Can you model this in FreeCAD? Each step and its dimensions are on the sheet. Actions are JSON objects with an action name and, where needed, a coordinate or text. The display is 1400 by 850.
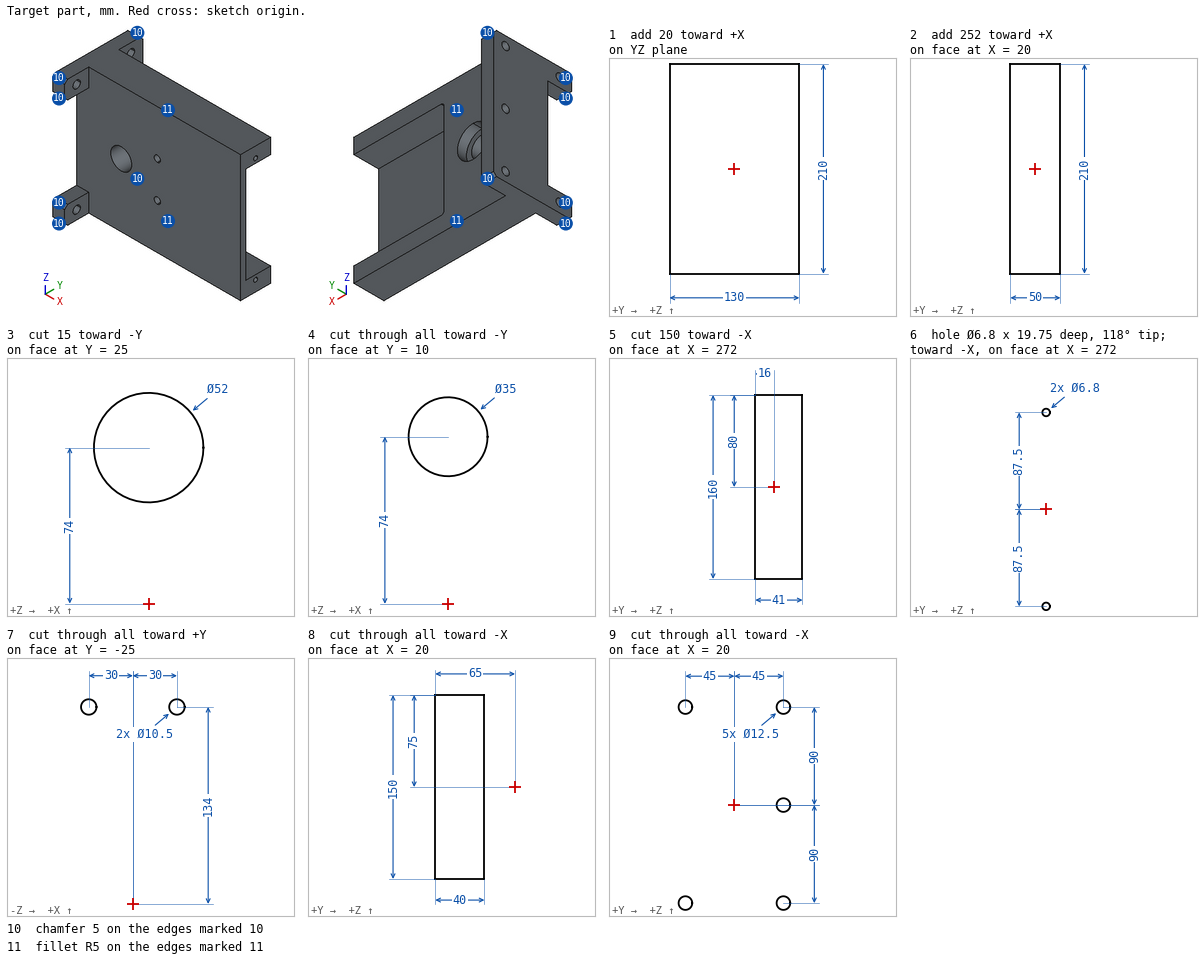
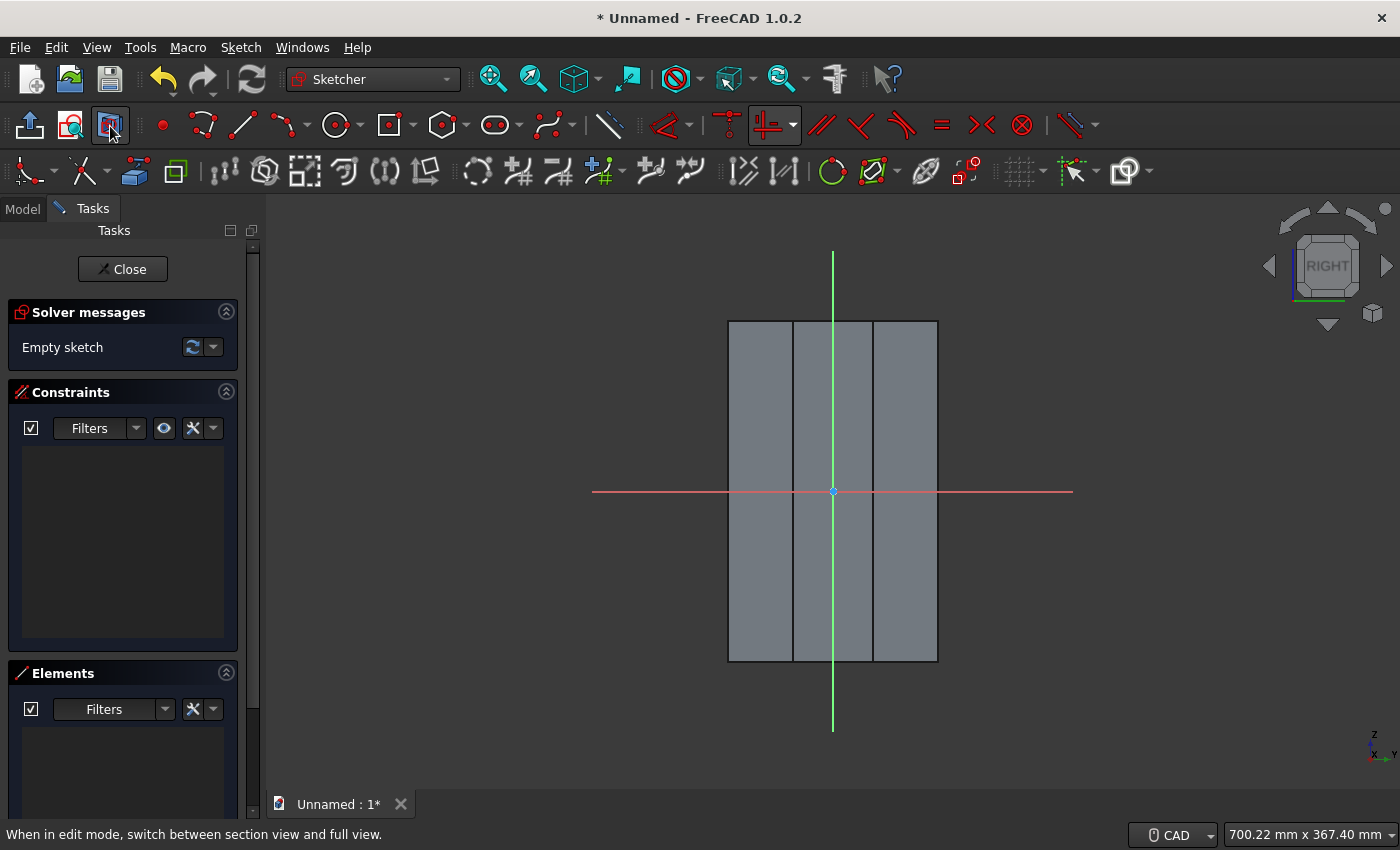
{"action": "scroll", "coordinate": [813, 492], "scroll_direction": "up", "scroll_amount": 2}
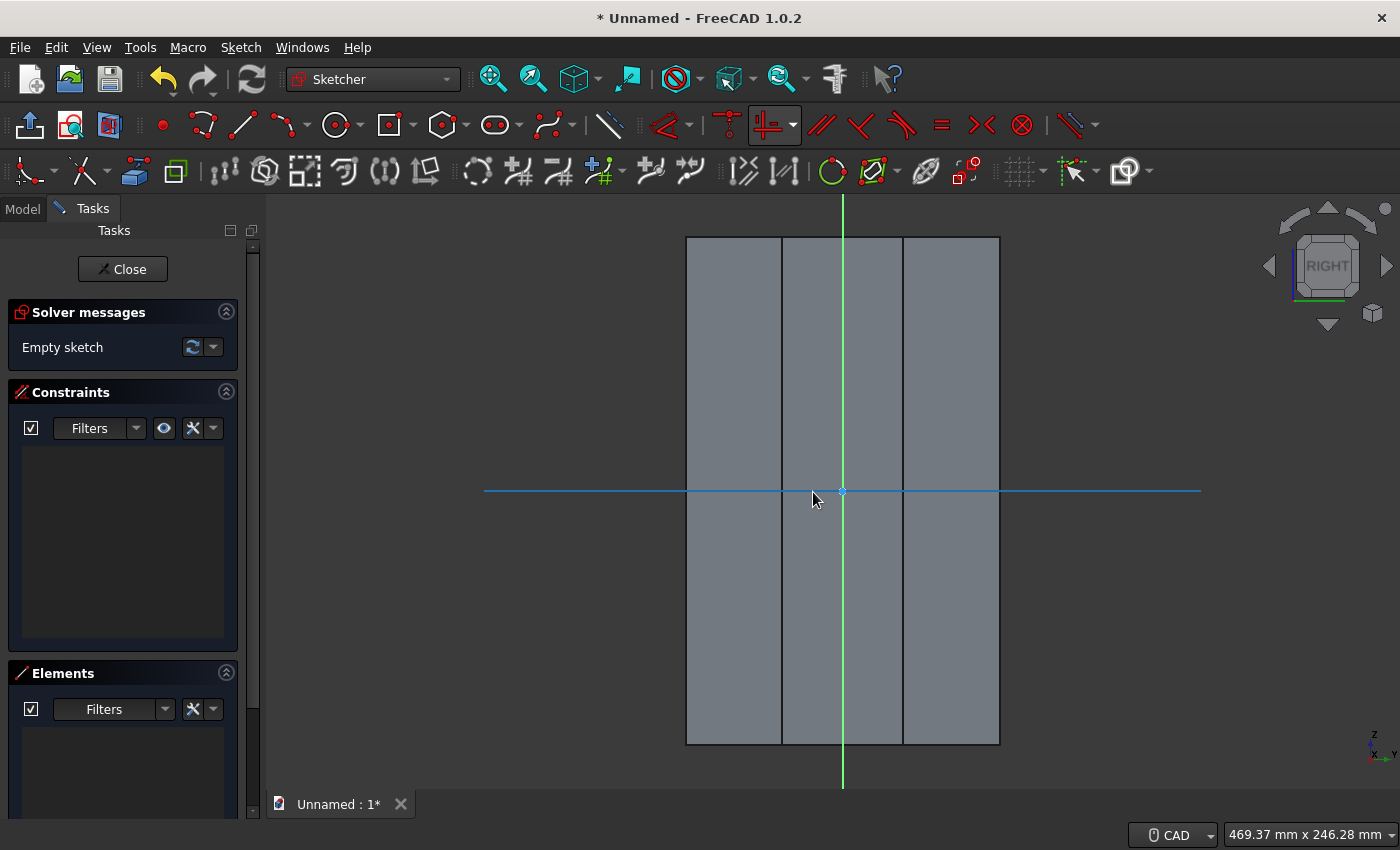
{"action": "left_click", "coordinate": [416, 126]}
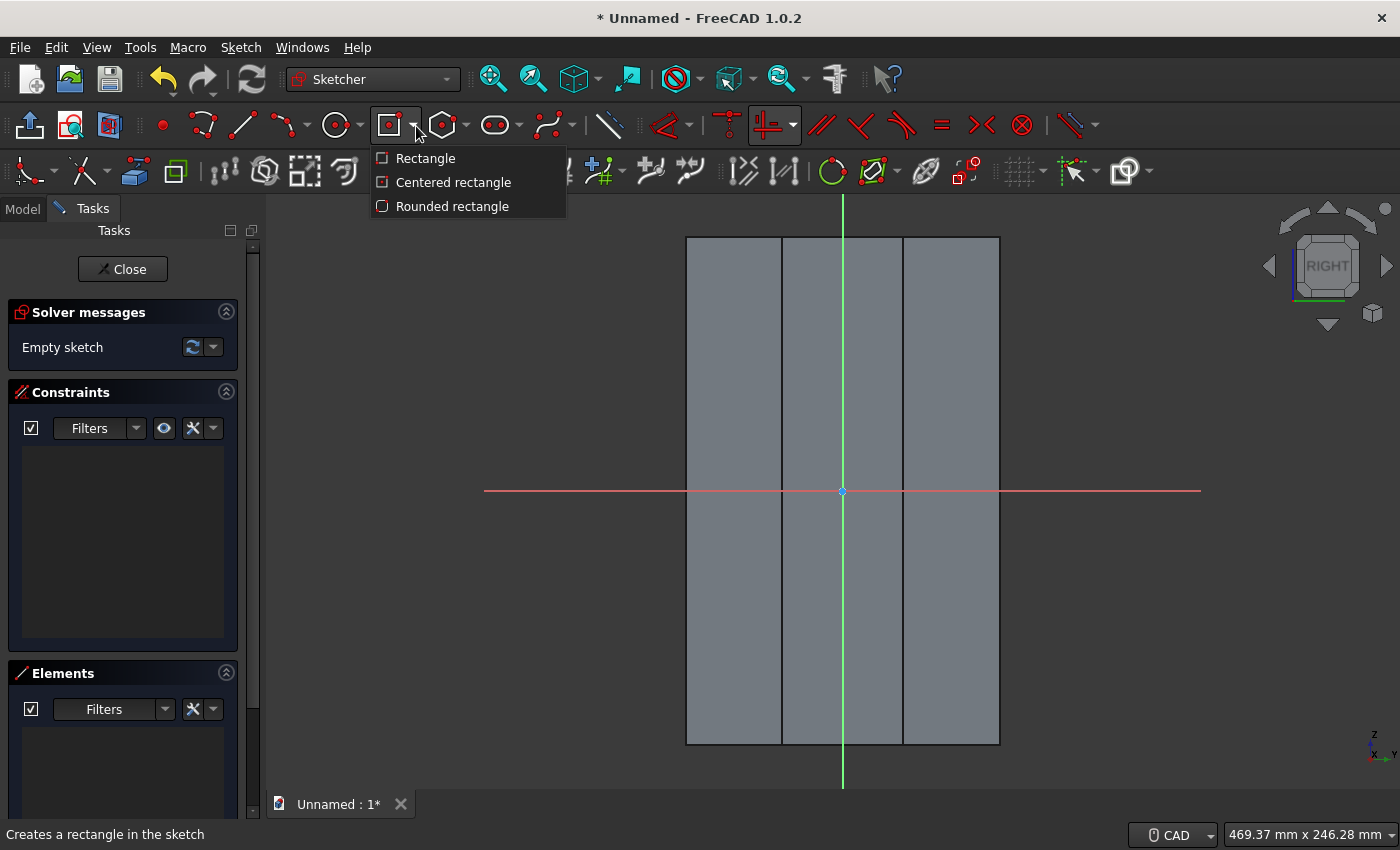
{"action": "left_click", "coordinate": [468, 158]}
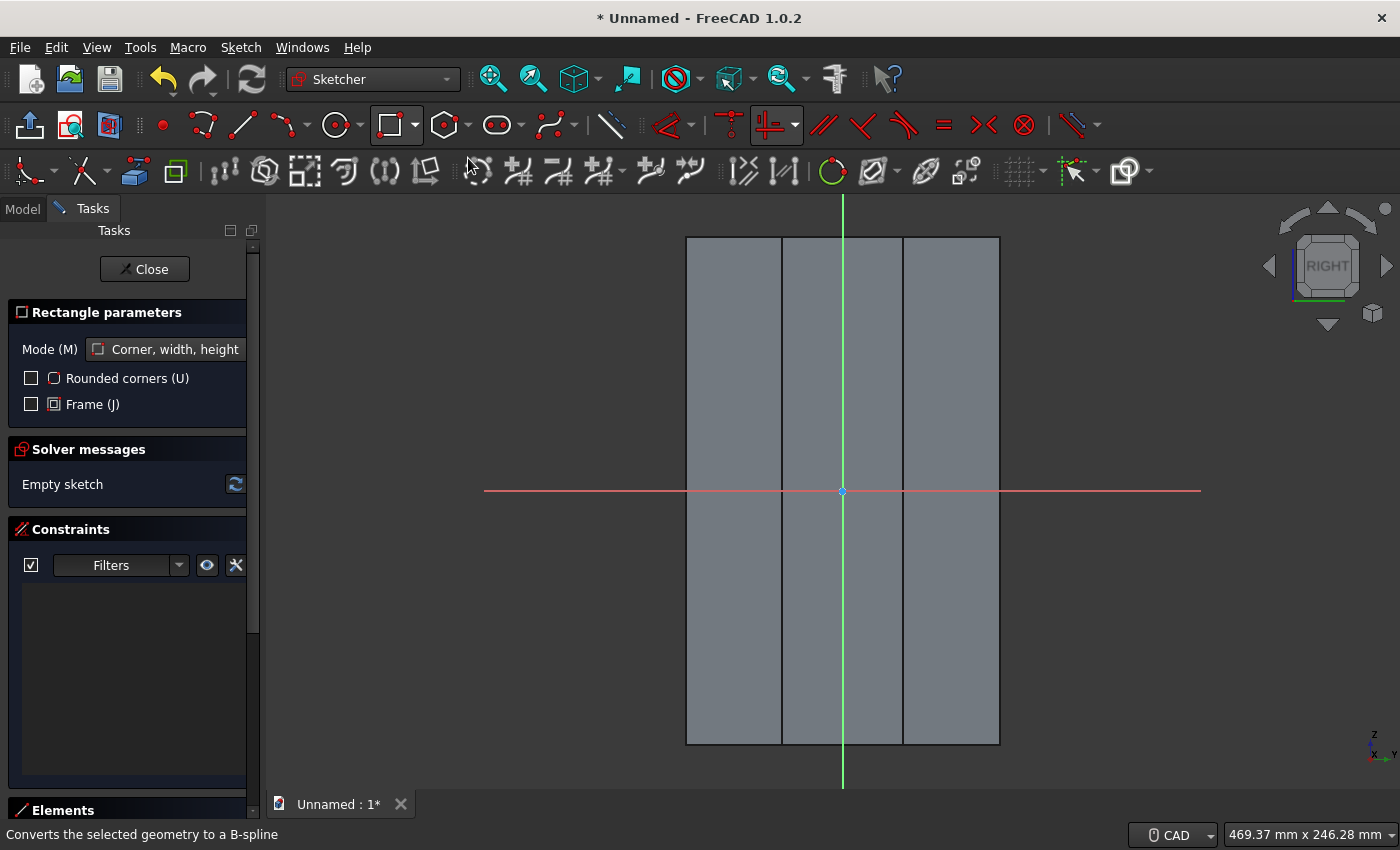
{"action": "left_click", "coordinate": [686, 310]}
{"action": "left_click", "coordinate": [782, 672]}
{"action": "key", "text": "Escape"}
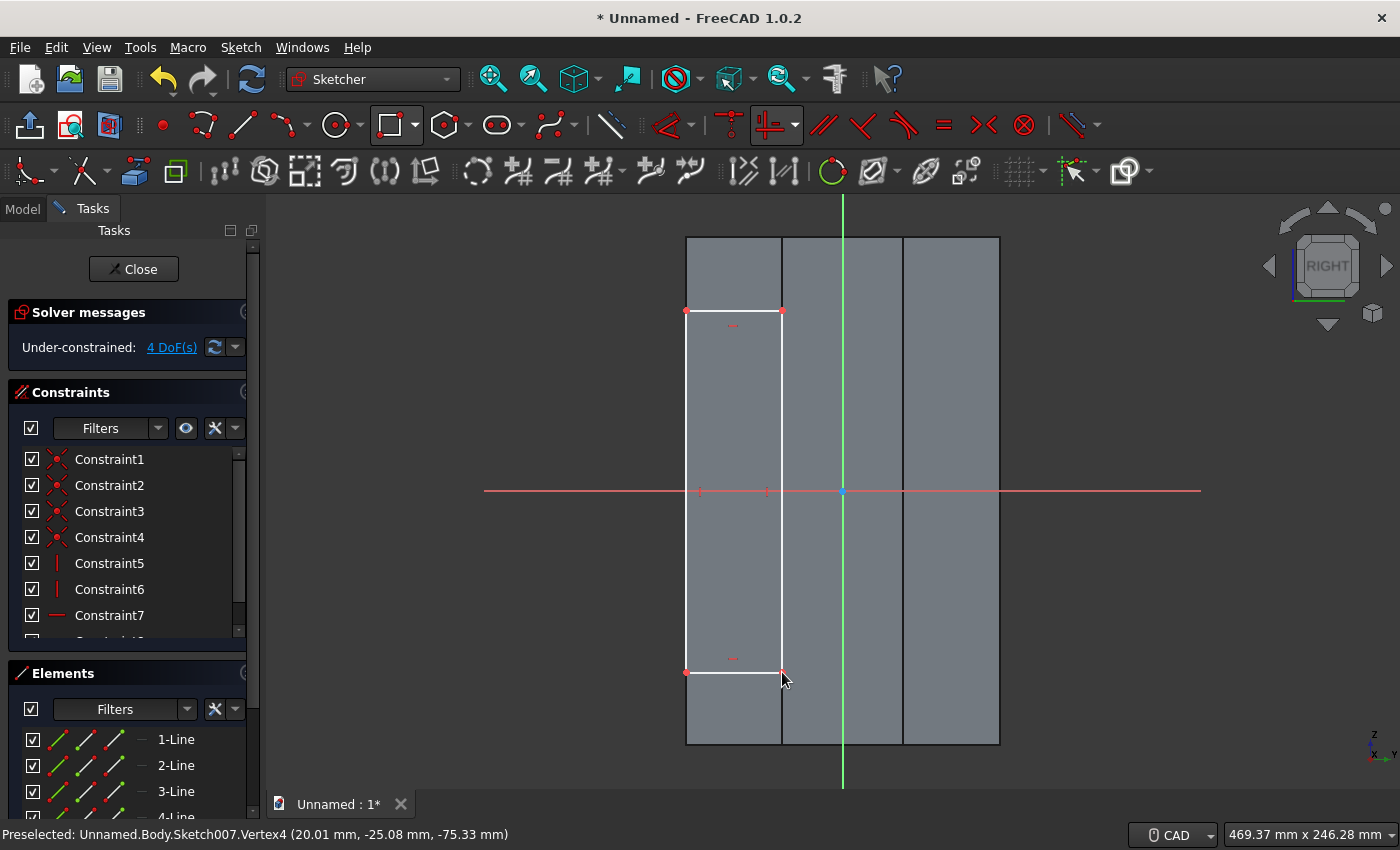
{"action": "left_click", "coordinate": [666, 126]}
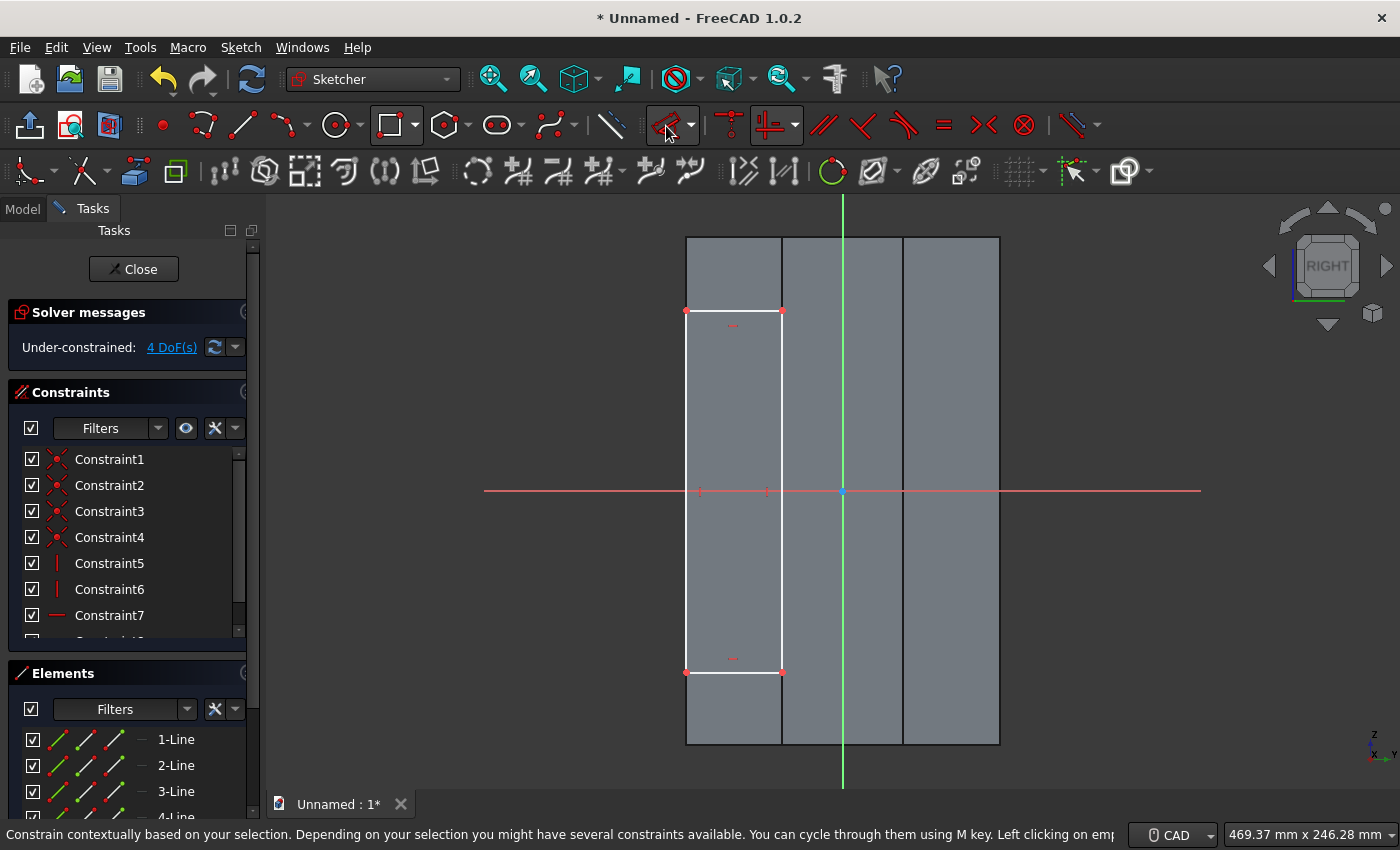
{"action": "left_click", "coordinate": [715, 673]}
{"action": "left_click", "coordinate": [734, 707]}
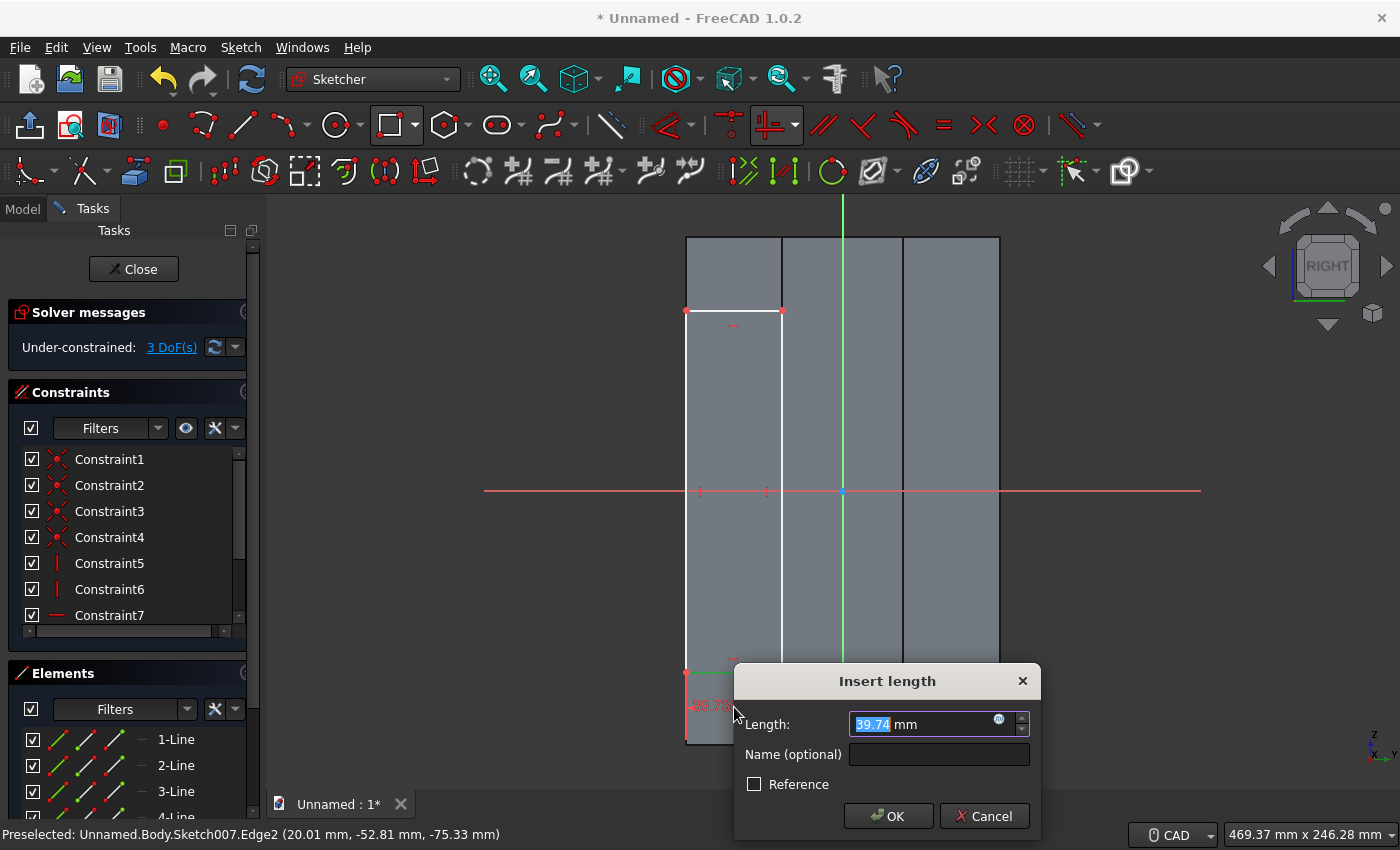
{"action": "type", "text": "40"}
{"action": "key", "text": "Return"}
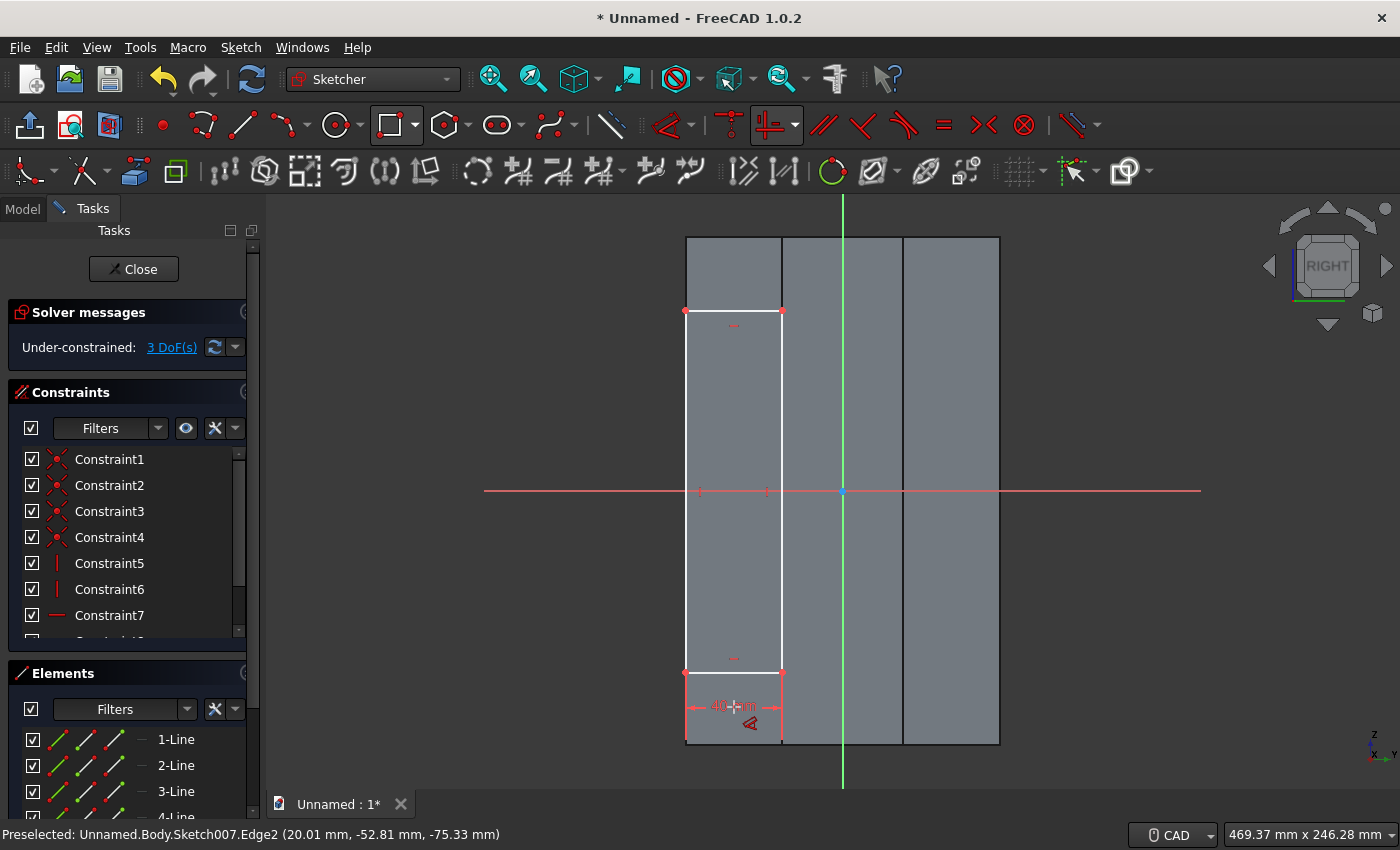
{"action": "left_click", "coordinate": [686, 420]}
{"action": "left_click", "coordinate": [652, 409]}